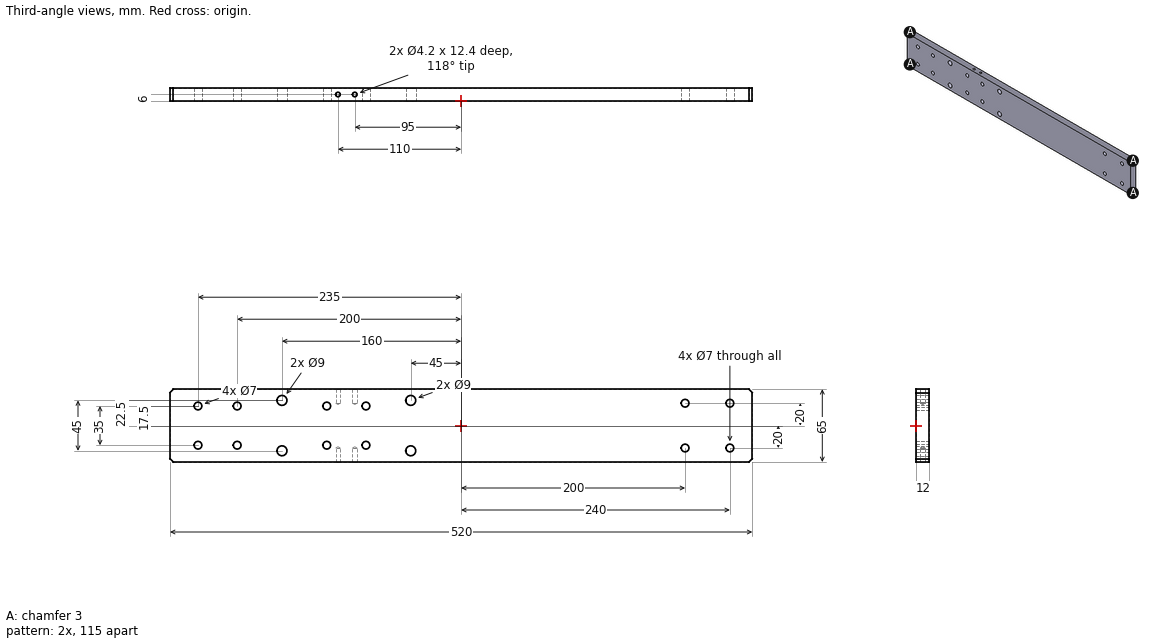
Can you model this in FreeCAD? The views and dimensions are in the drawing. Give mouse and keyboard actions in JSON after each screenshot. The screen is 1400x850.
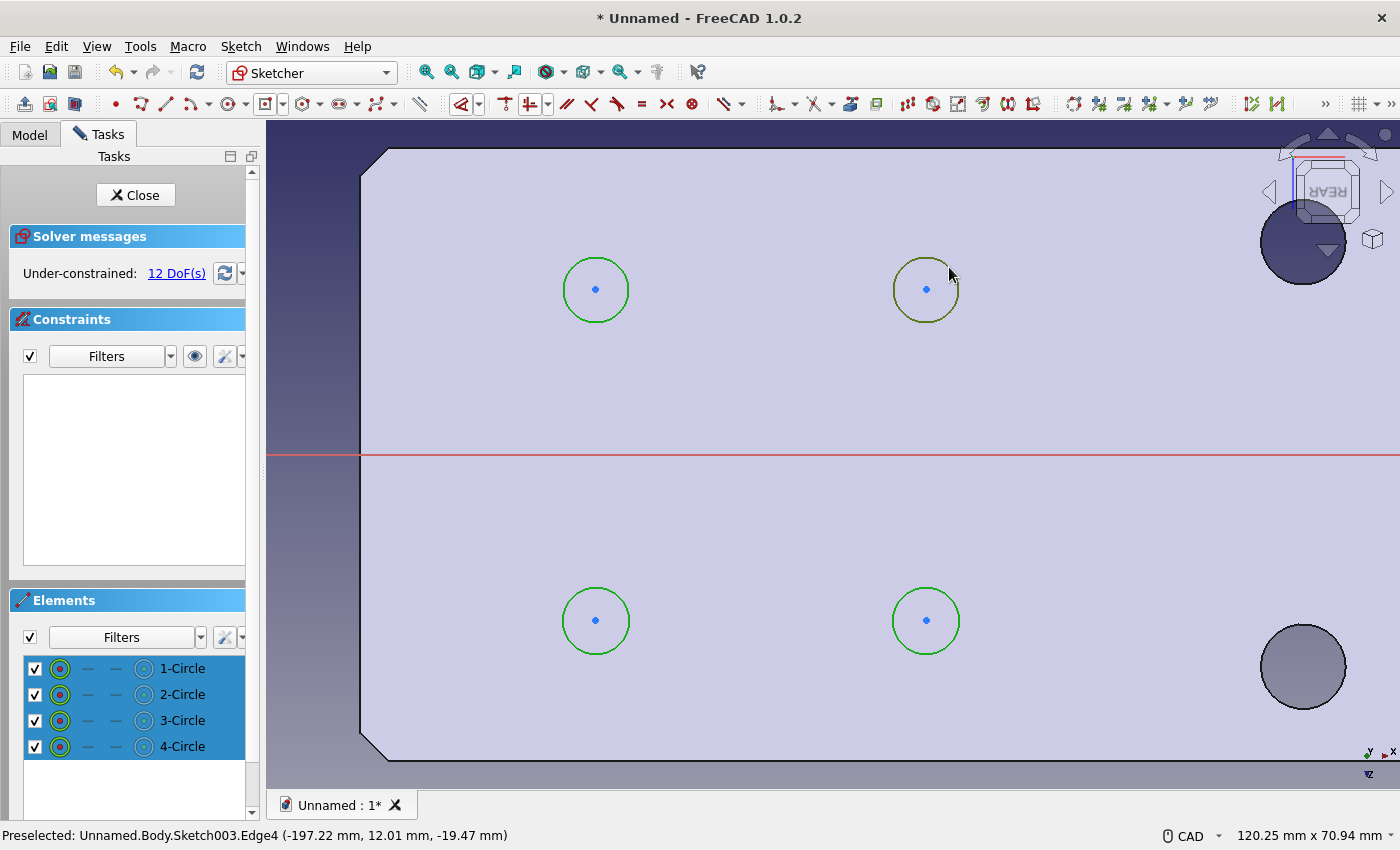
{"action": "left_click", "coordinate": [642, 104]}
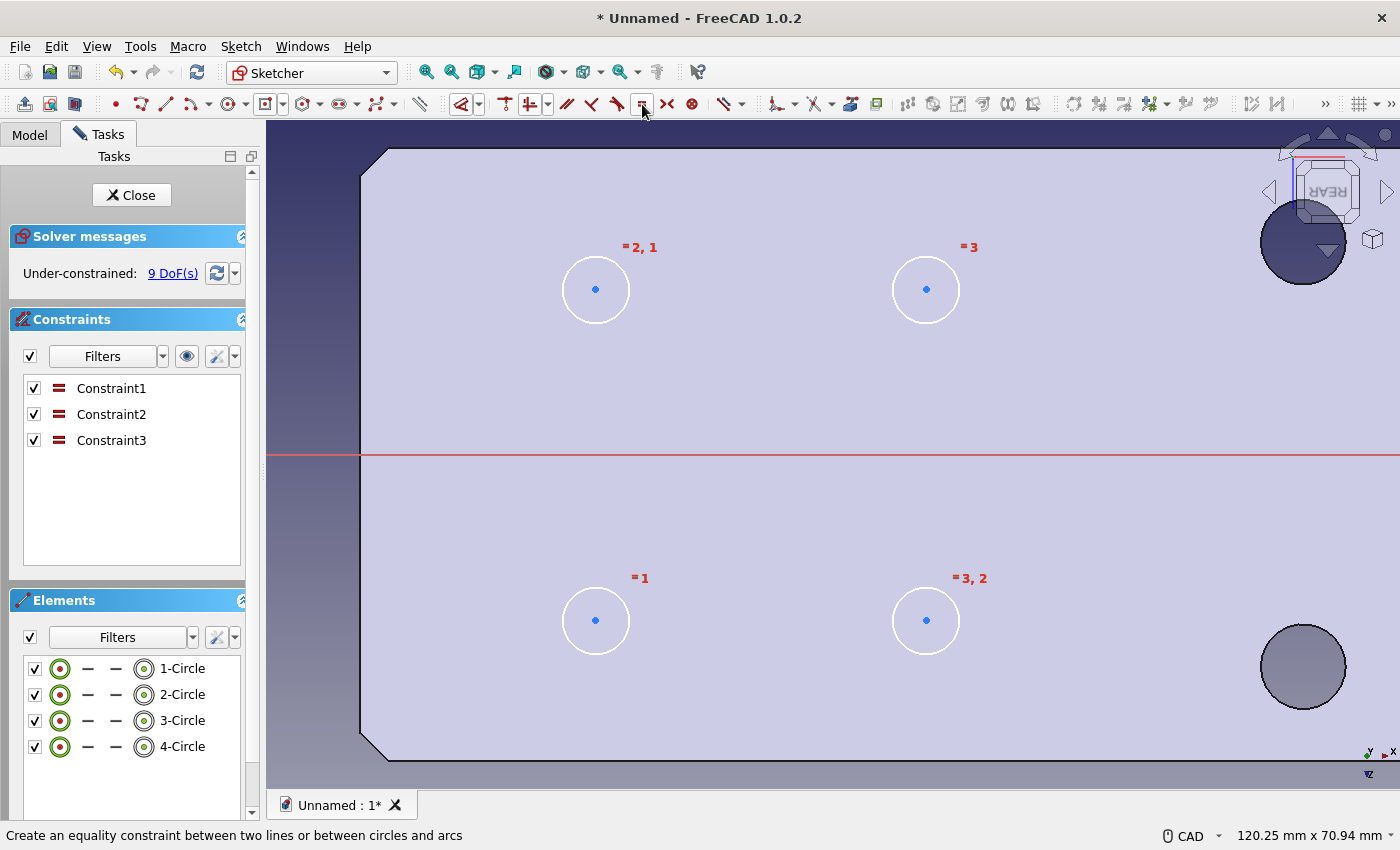
{"action": "left_click", "coordinate": [596, 621]}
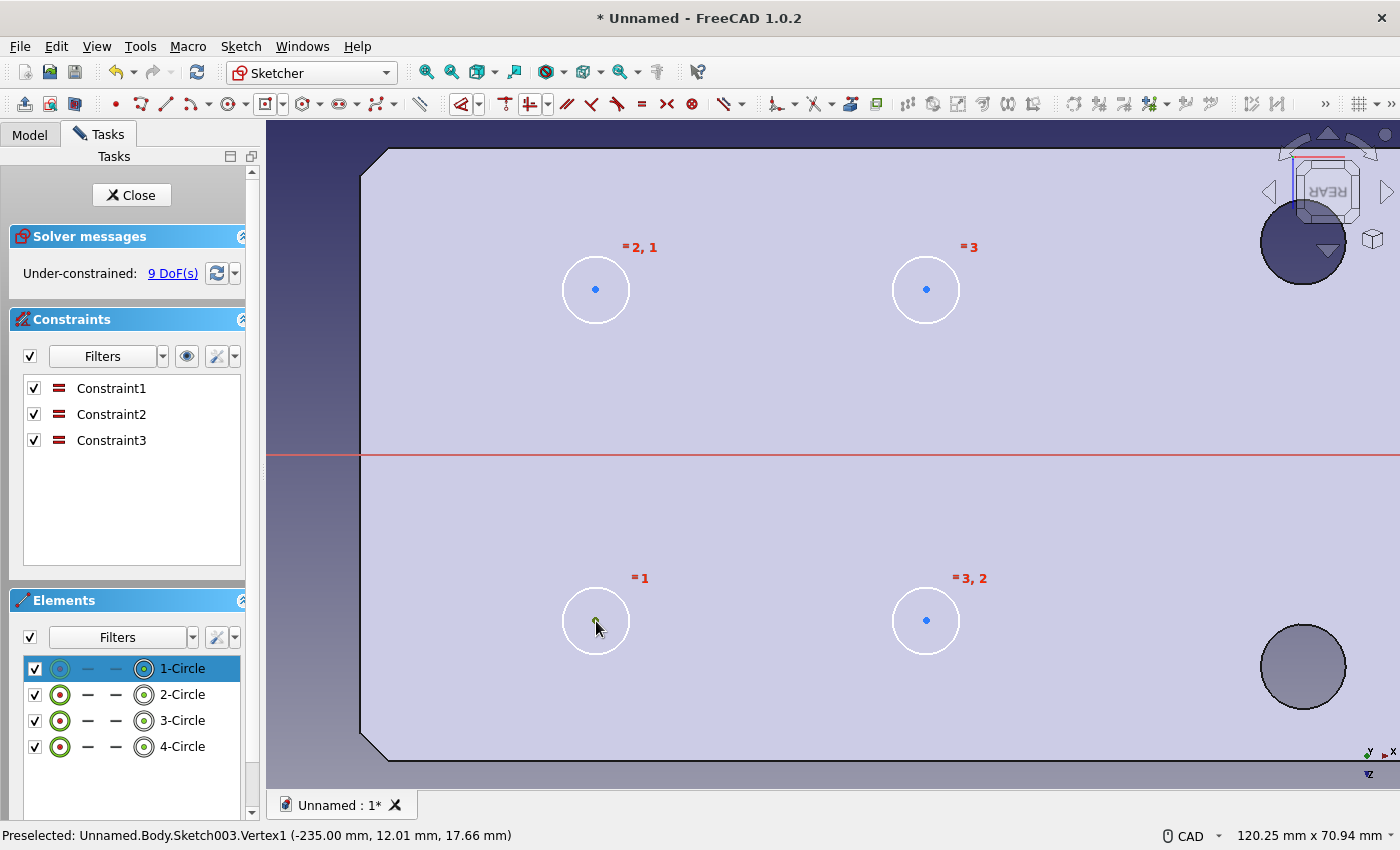
{"action": "left_click", "coordinate": [596, 290]}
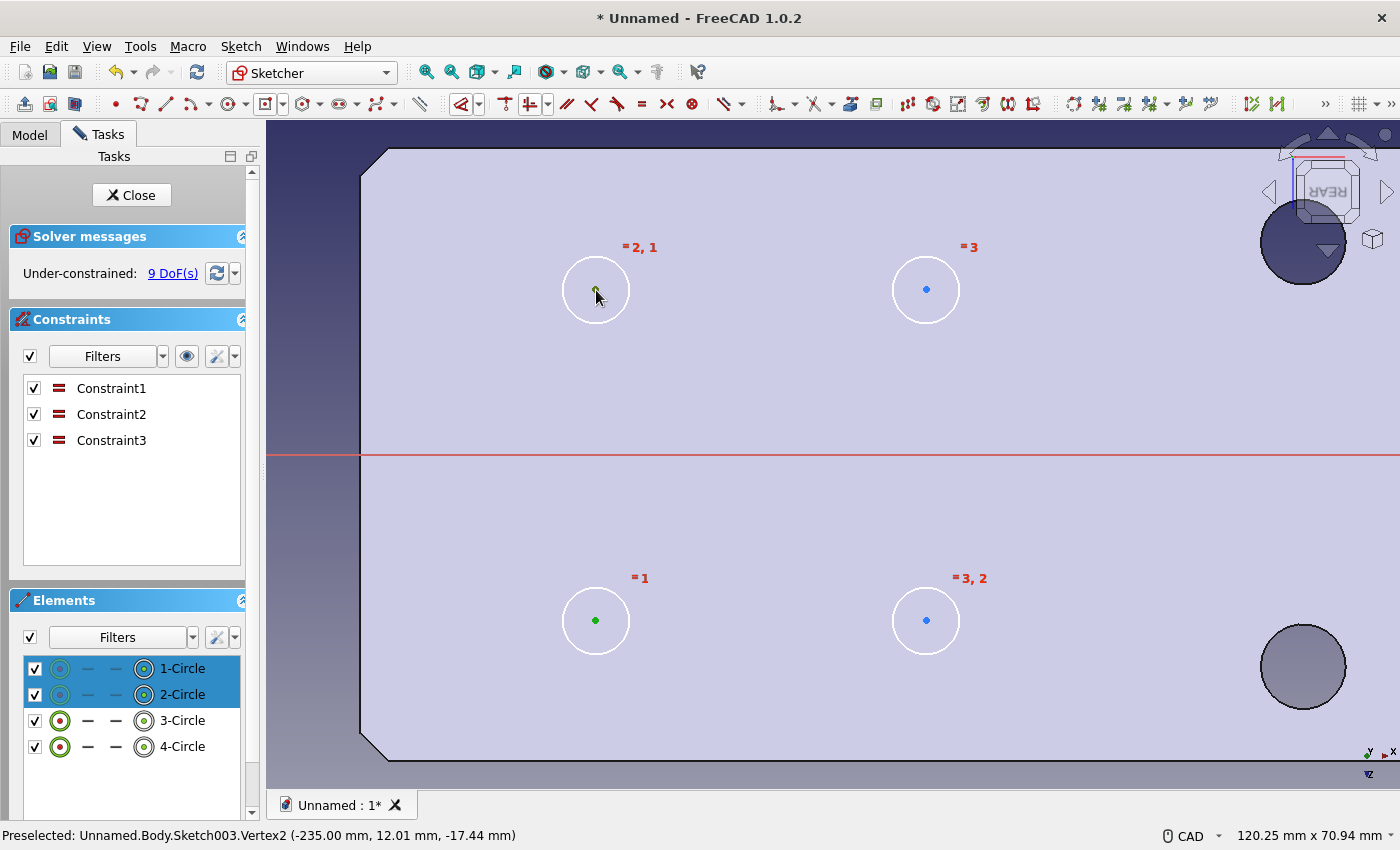
{"action": "key", "text": "v"}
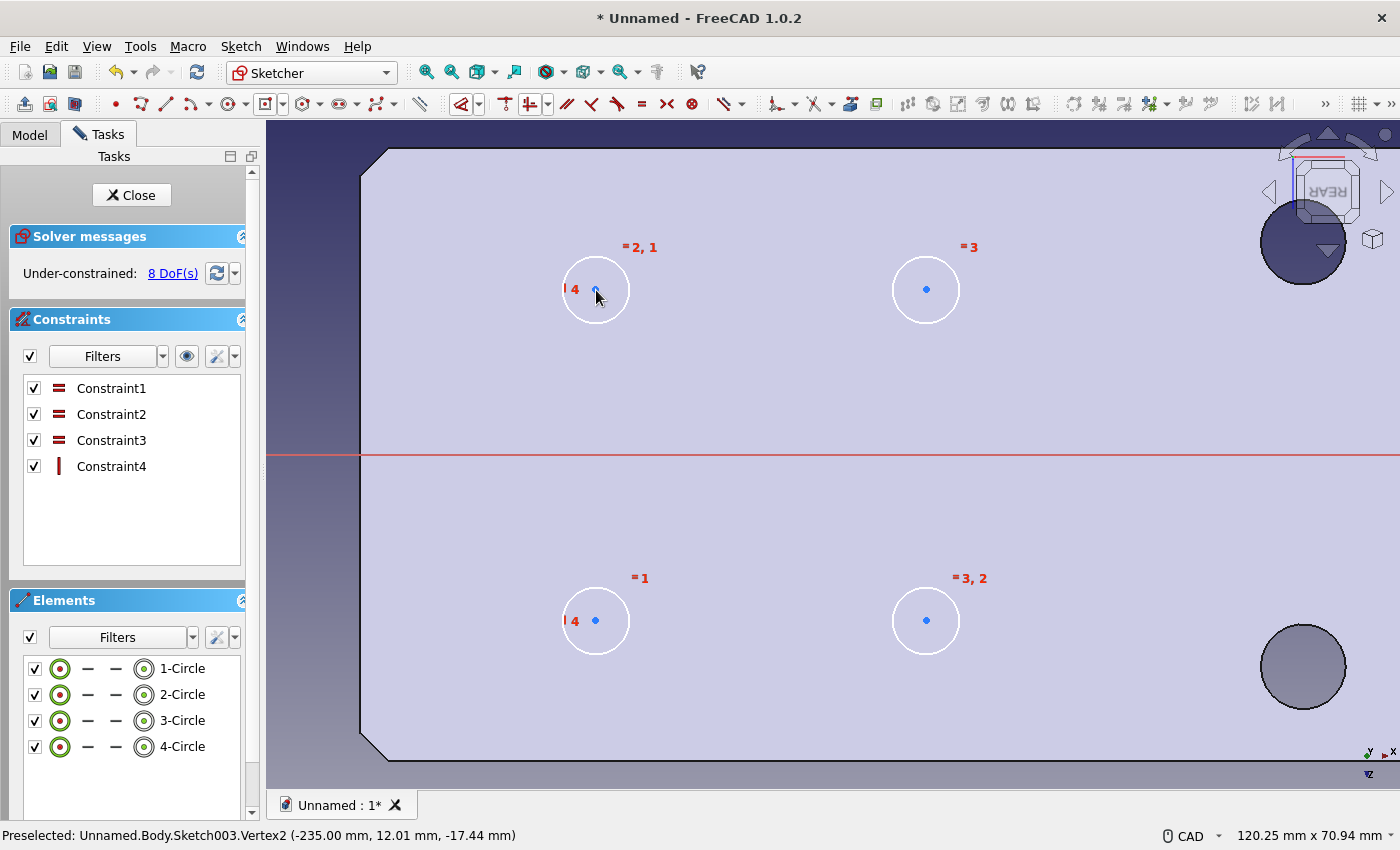
{"action": "left_click", "coordinate": [596, 621]}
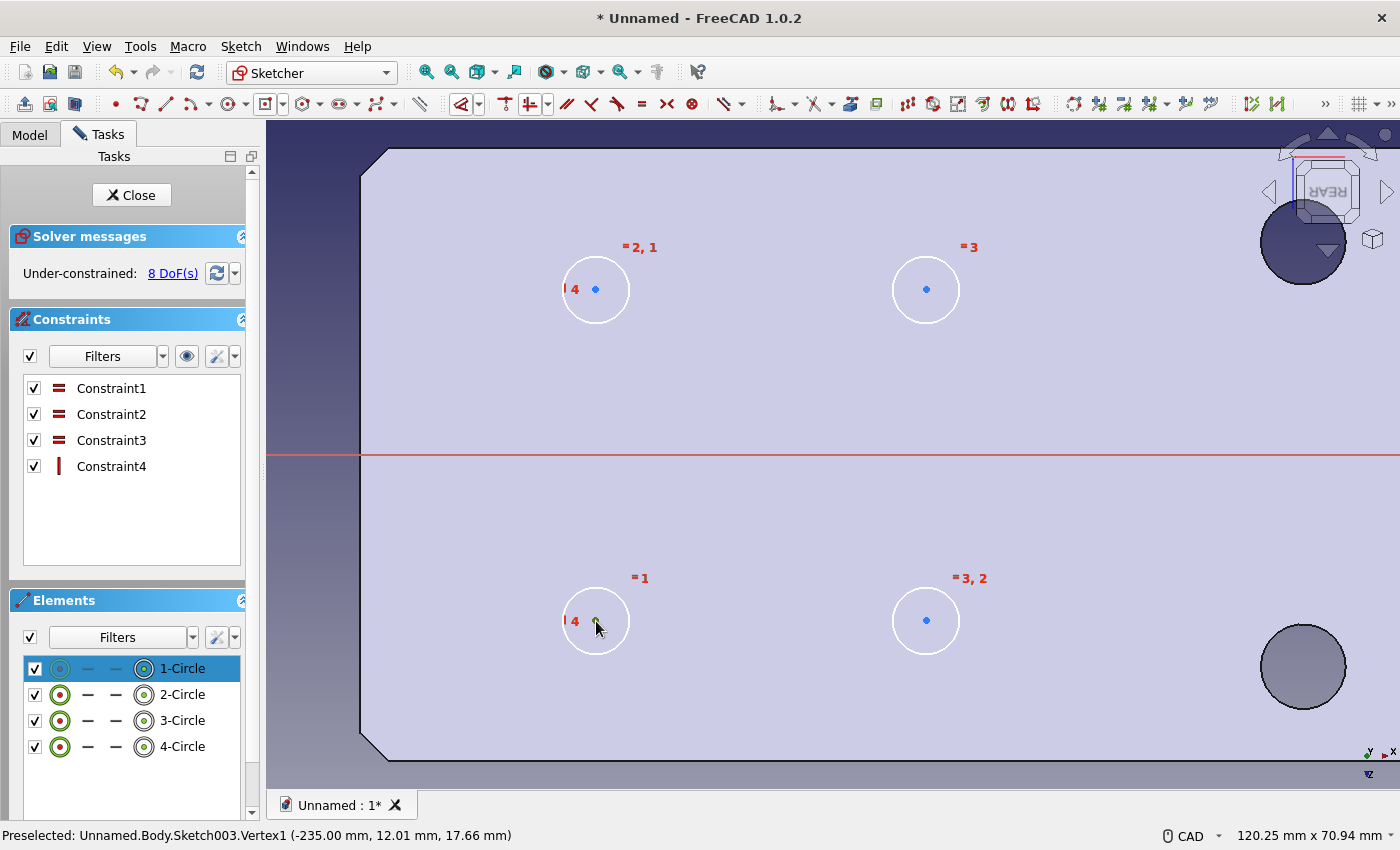
{"action": "left_click", "coordinate": [926, 621]}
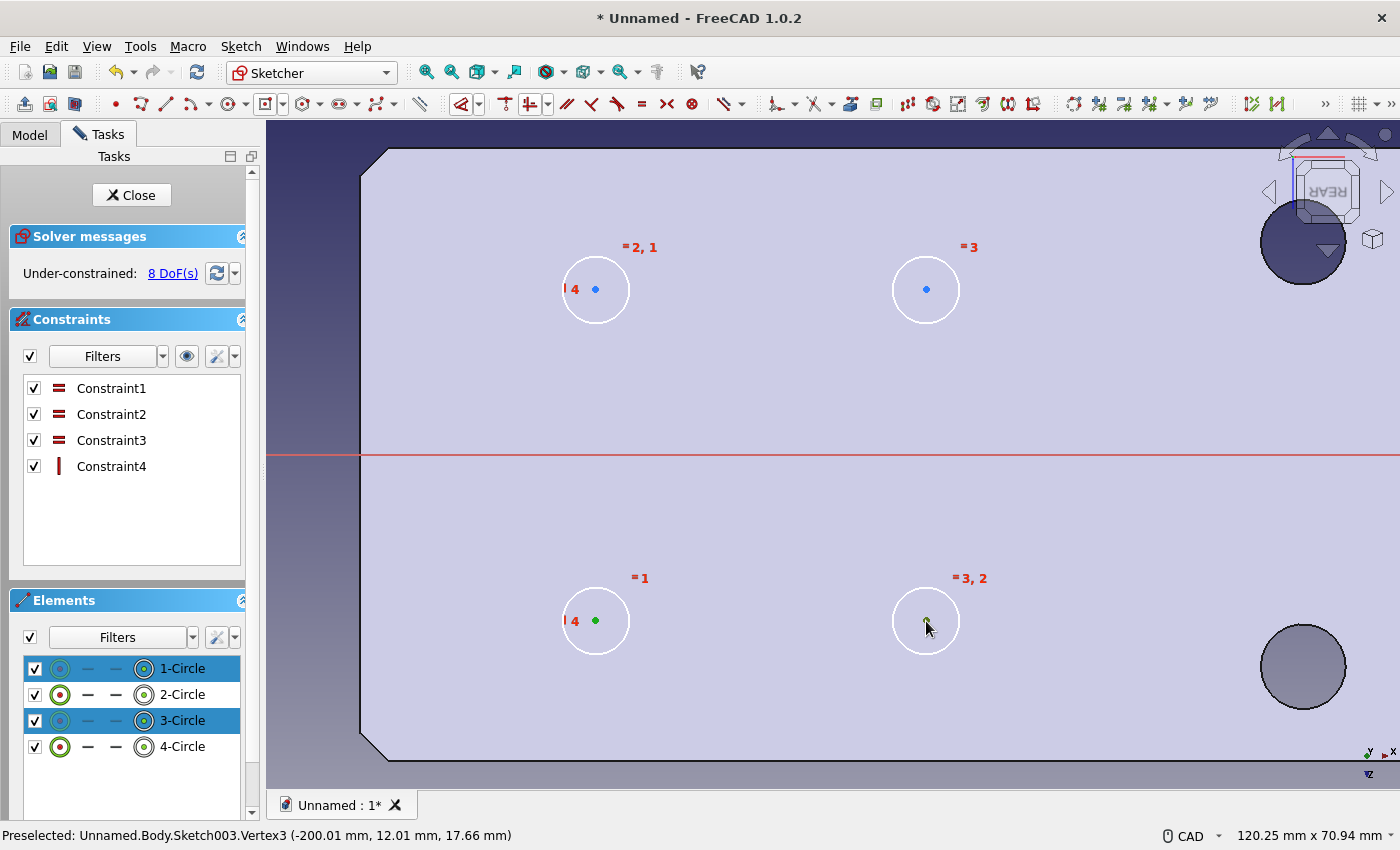
{"action": "left_click", "coordinate": [548, 104]}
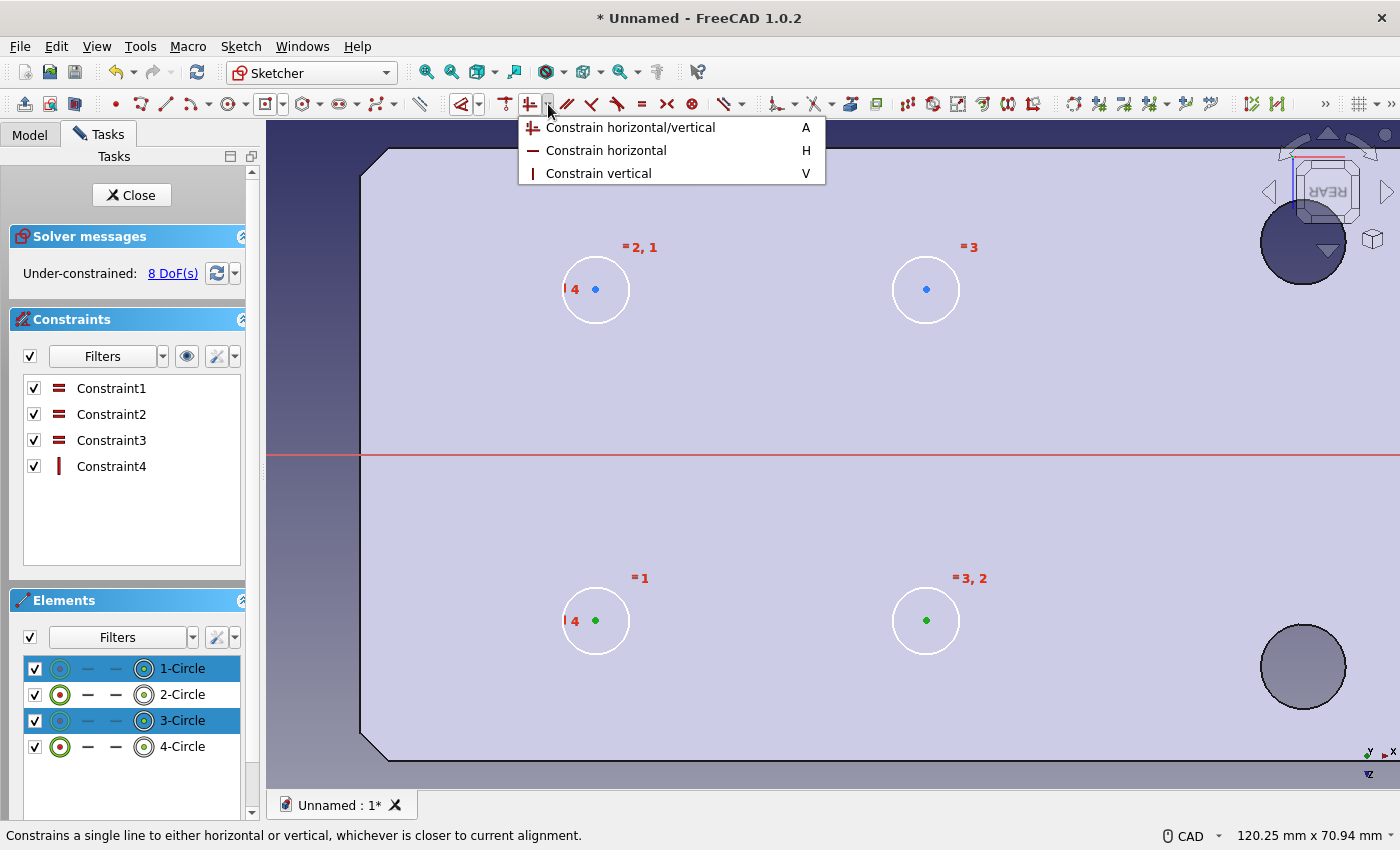
{"action": "left_click", "coordinate": [672, 150]}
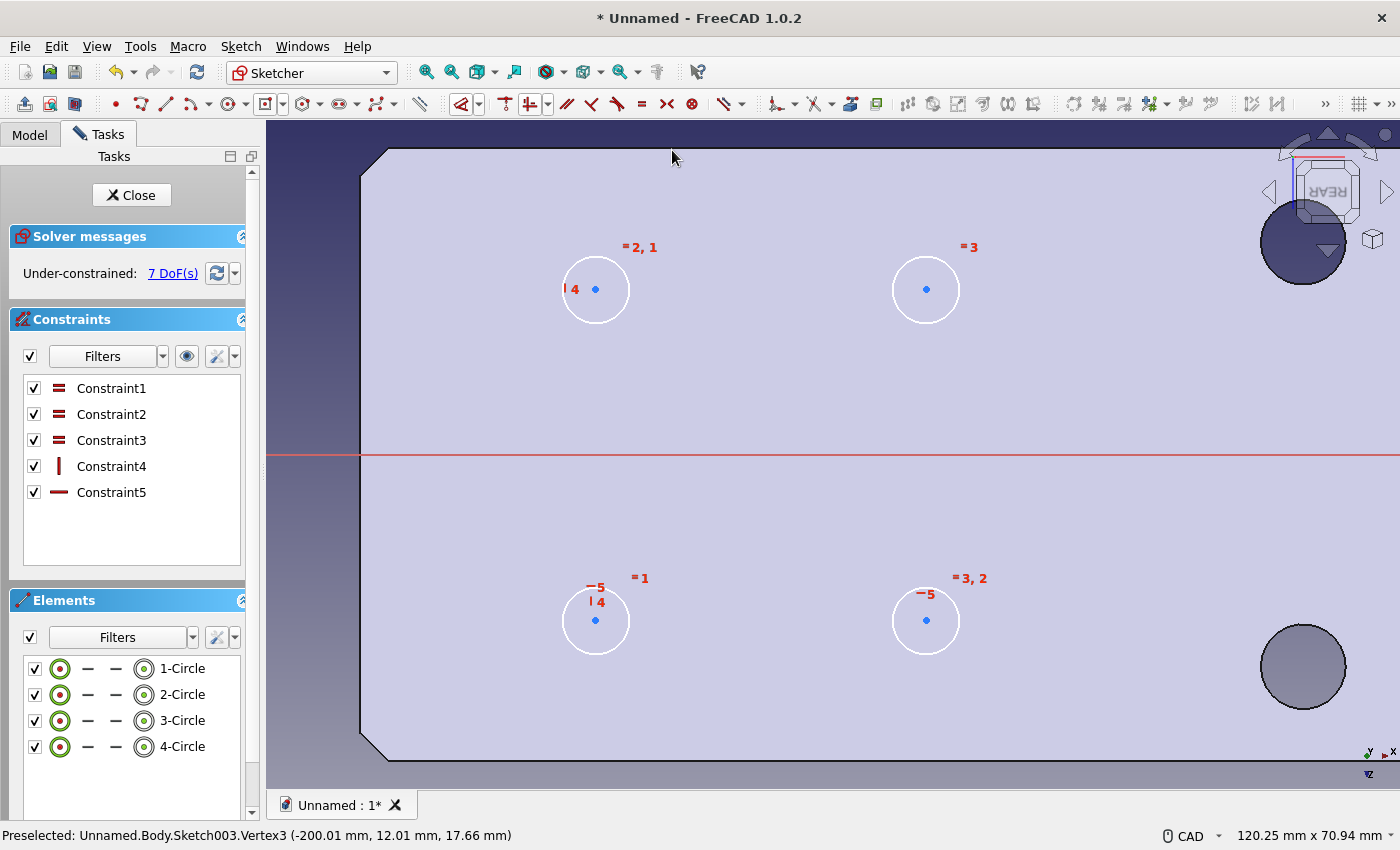
{"action": "left_click", "coordinate": [926, 621]}